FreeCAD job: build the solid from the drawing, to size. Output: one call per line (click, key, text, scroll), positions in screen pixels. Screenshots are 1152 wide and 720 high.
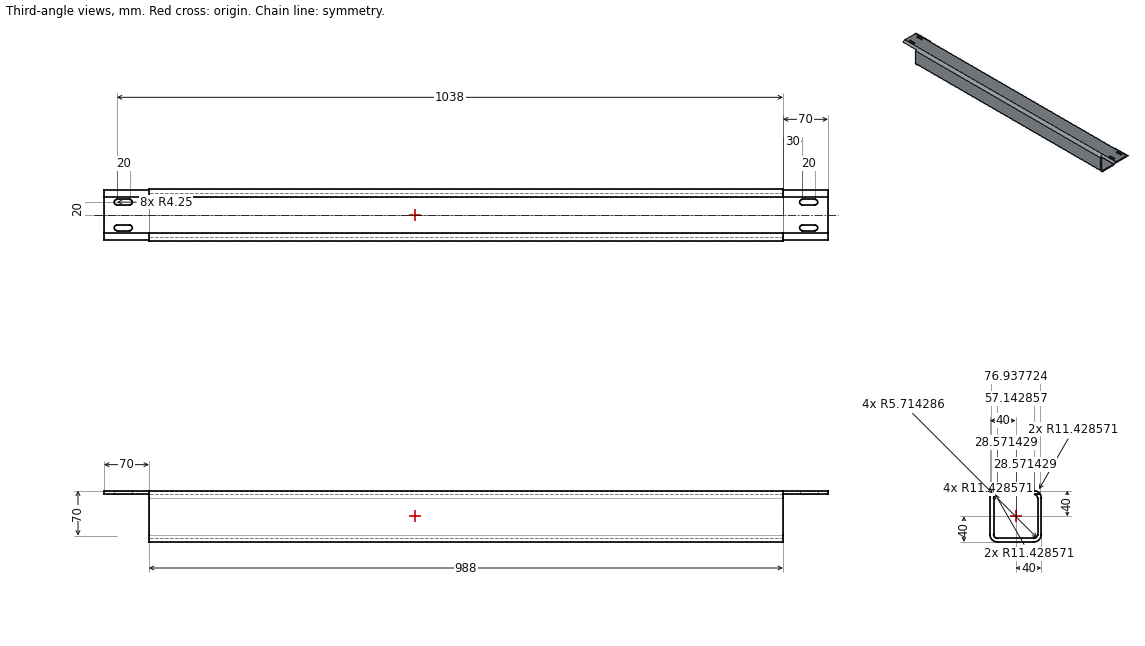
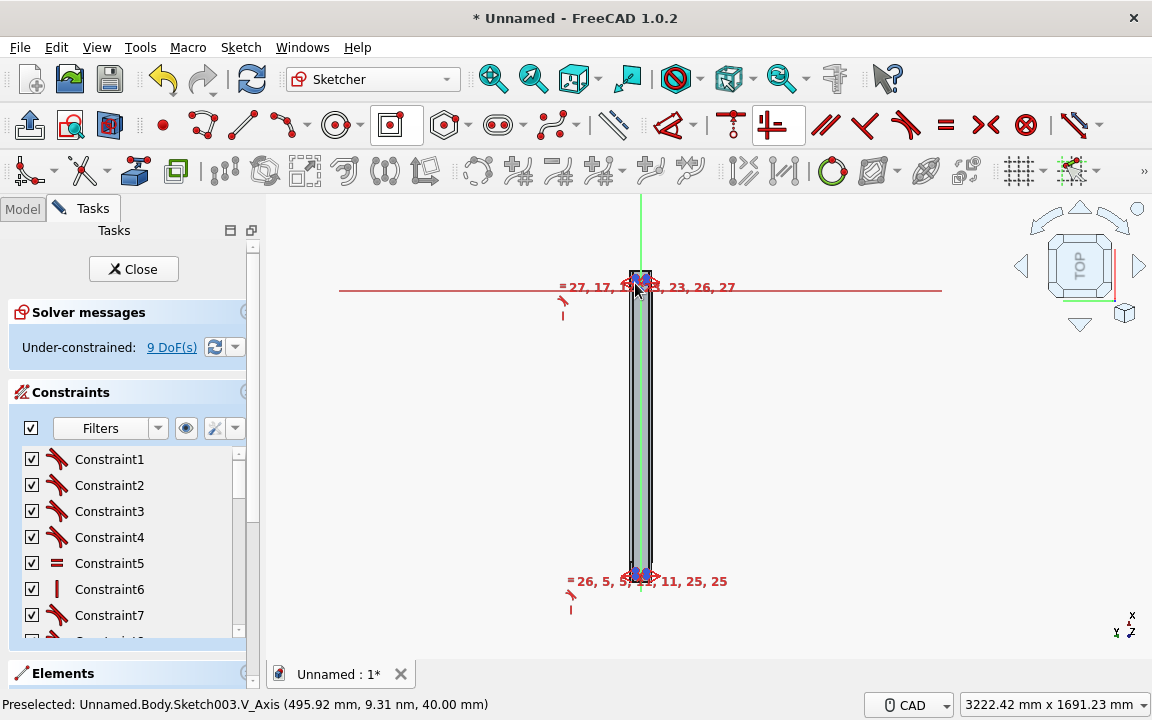
scroll(635, 577, up, 18)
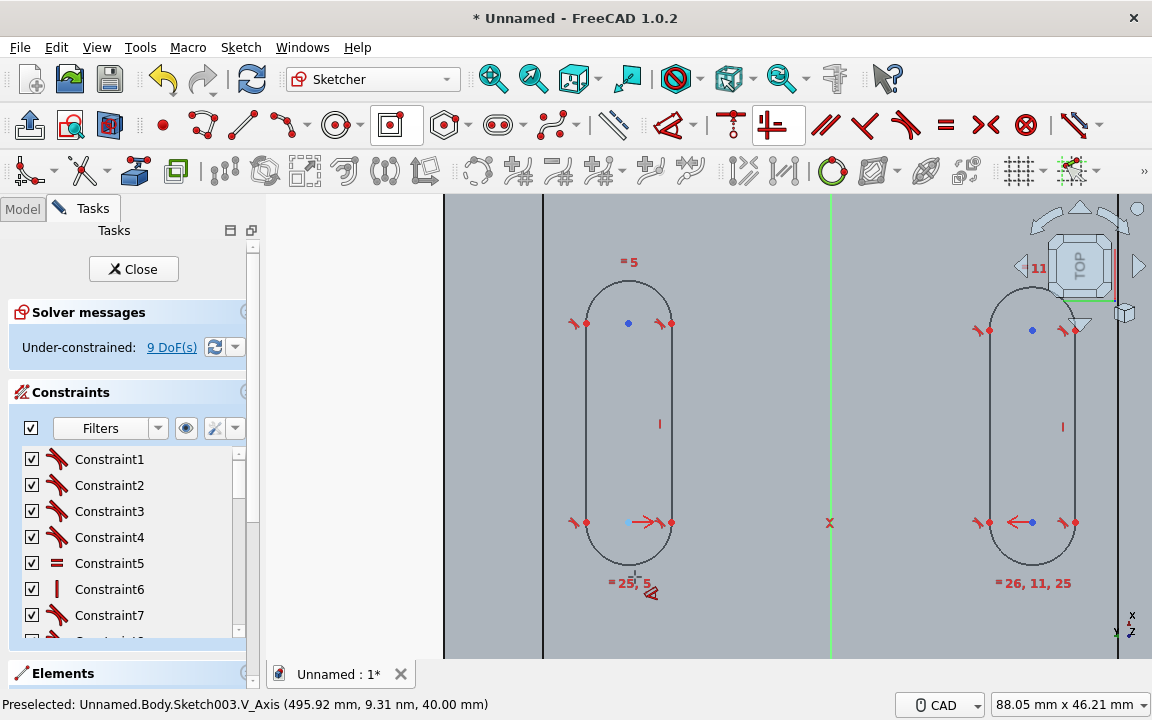
click(604, 557)
click(585, 583)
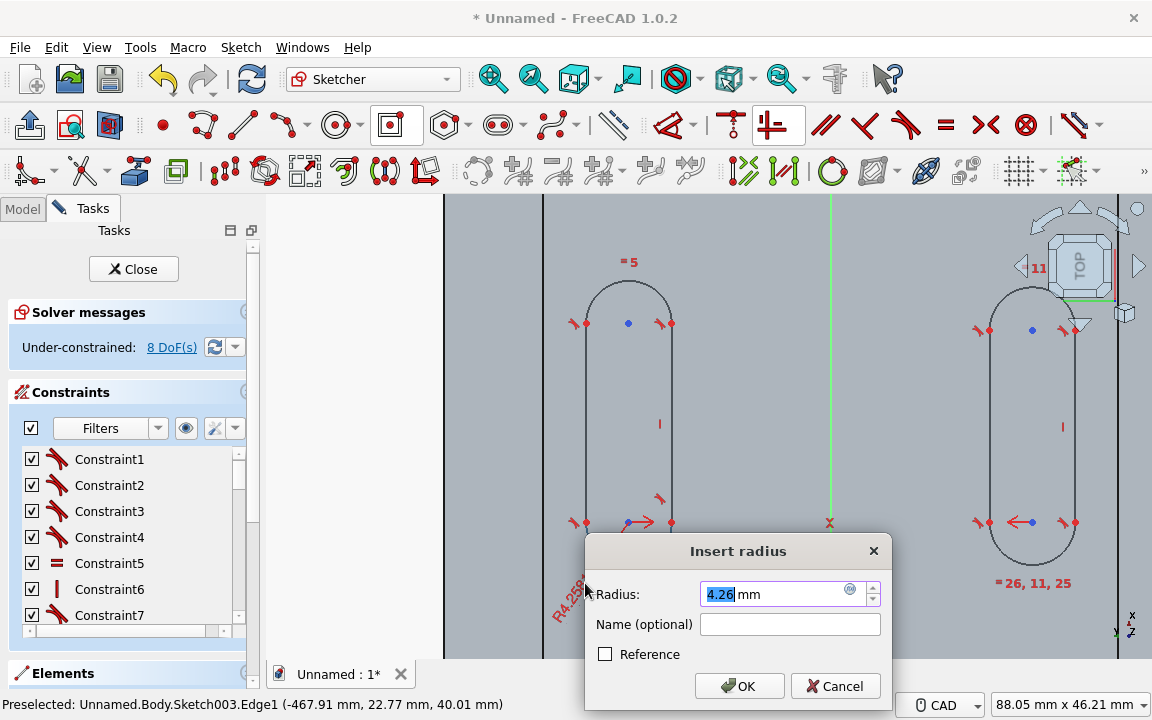
text(4.25)
key(Return)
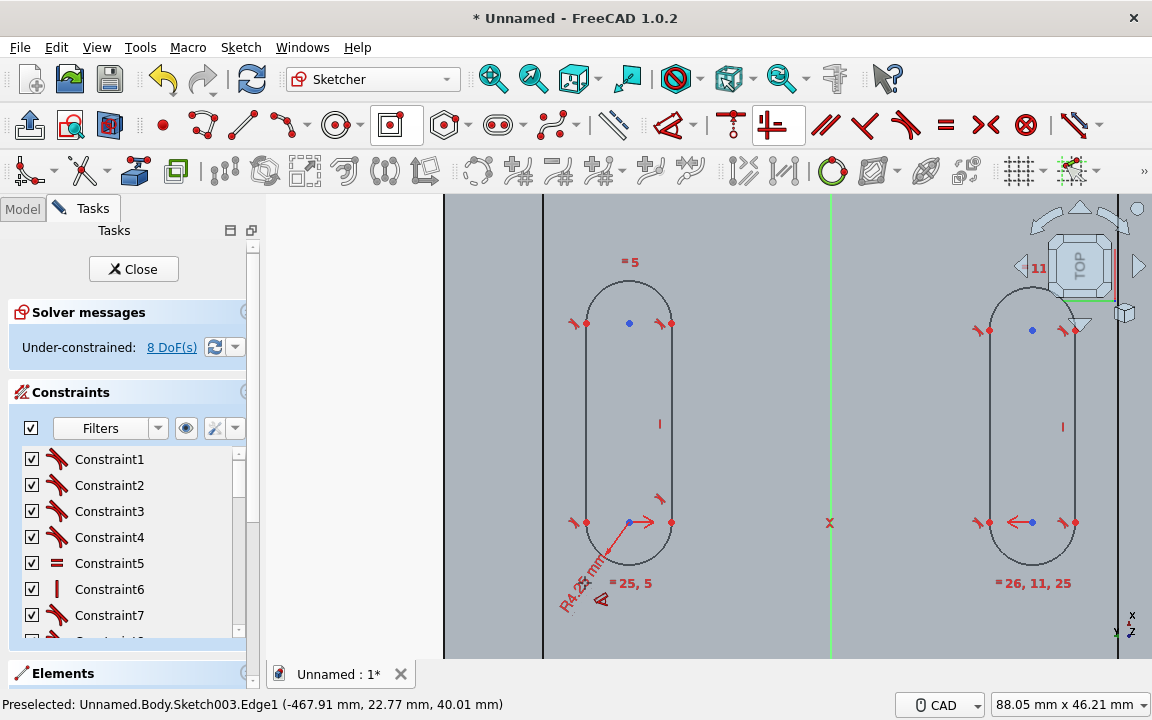
scroll(635, 578, down, 18)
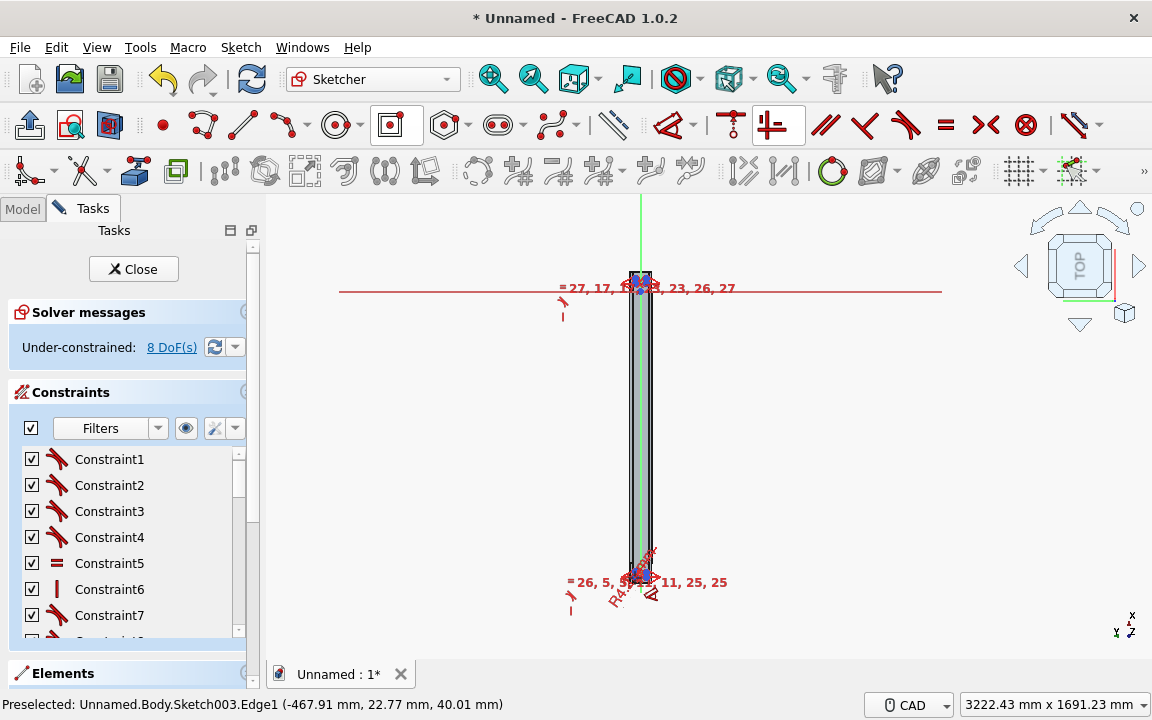
scroll(634, 576, up, 11)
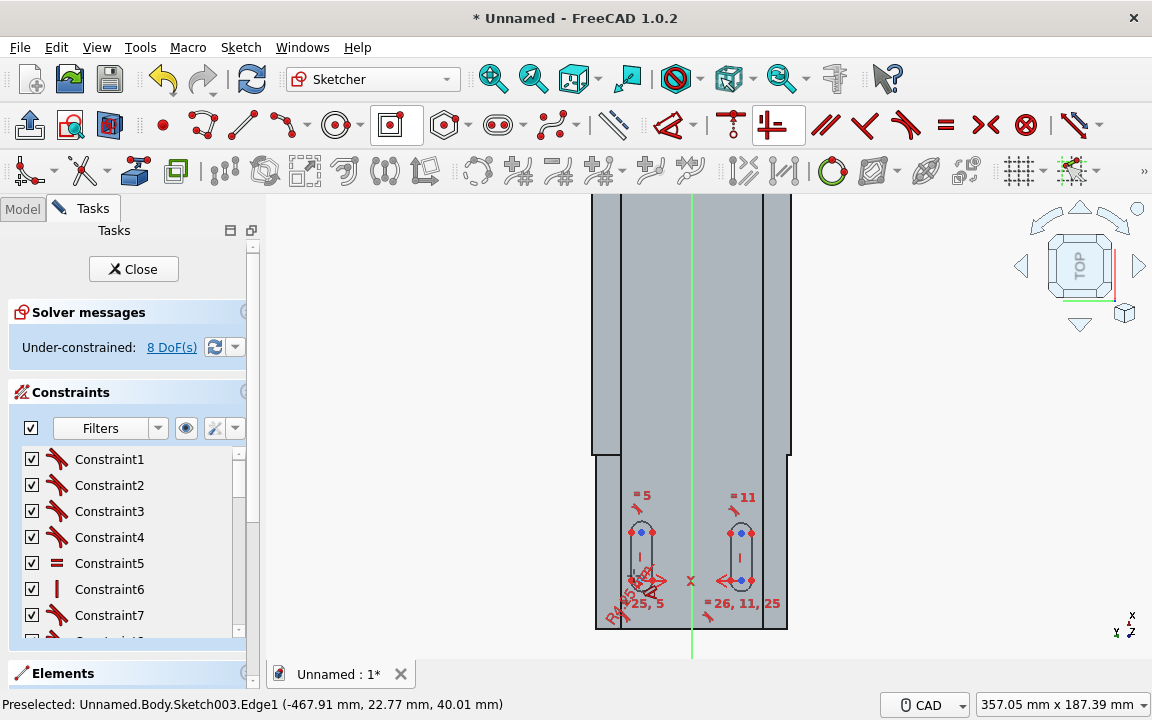
click(631, 566)
click(597, 556)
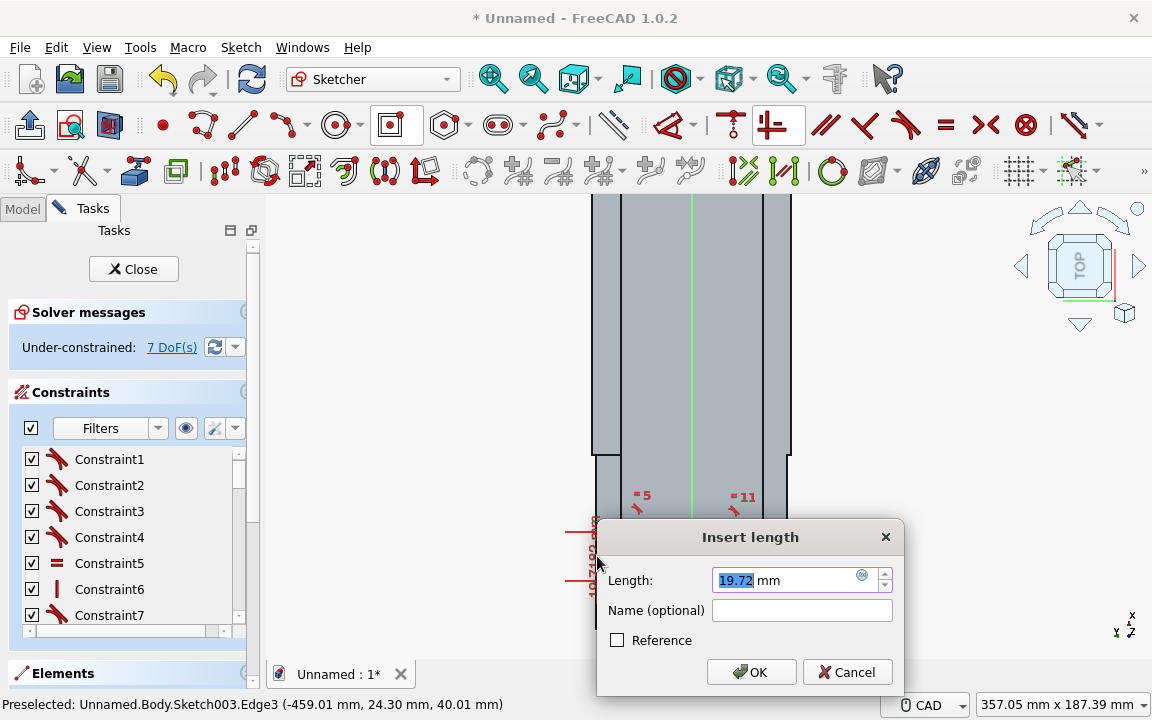
text(20)
key(Return)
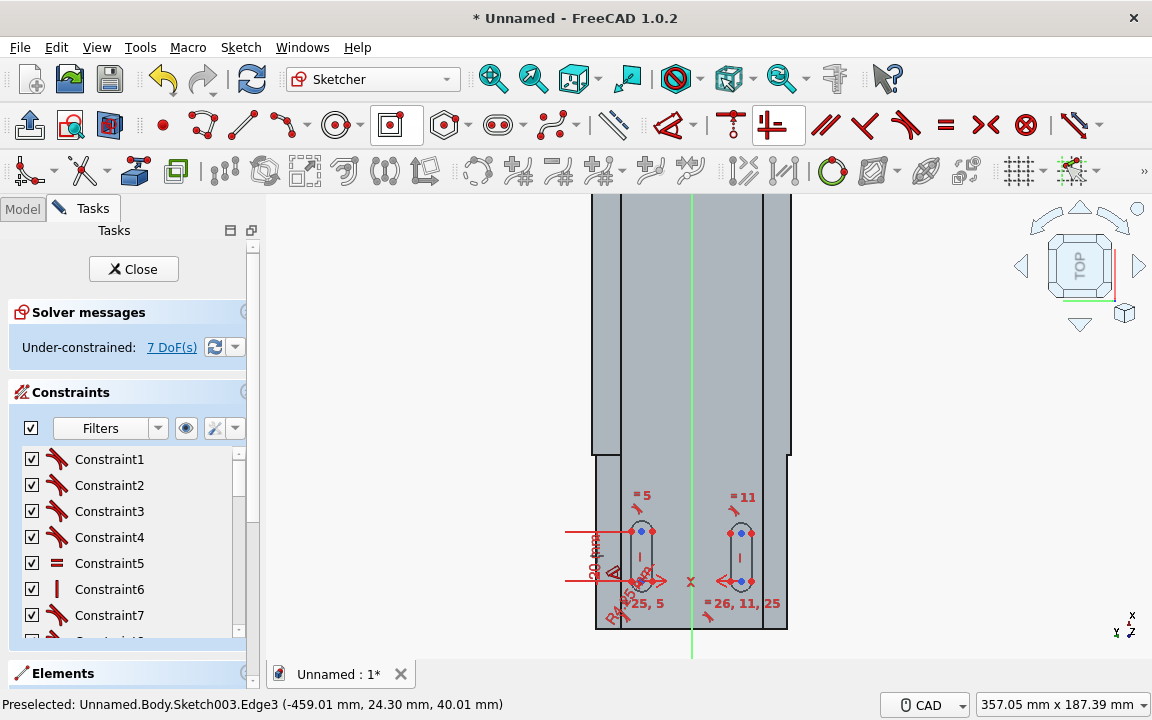
click(731, 567)
click(789, 557)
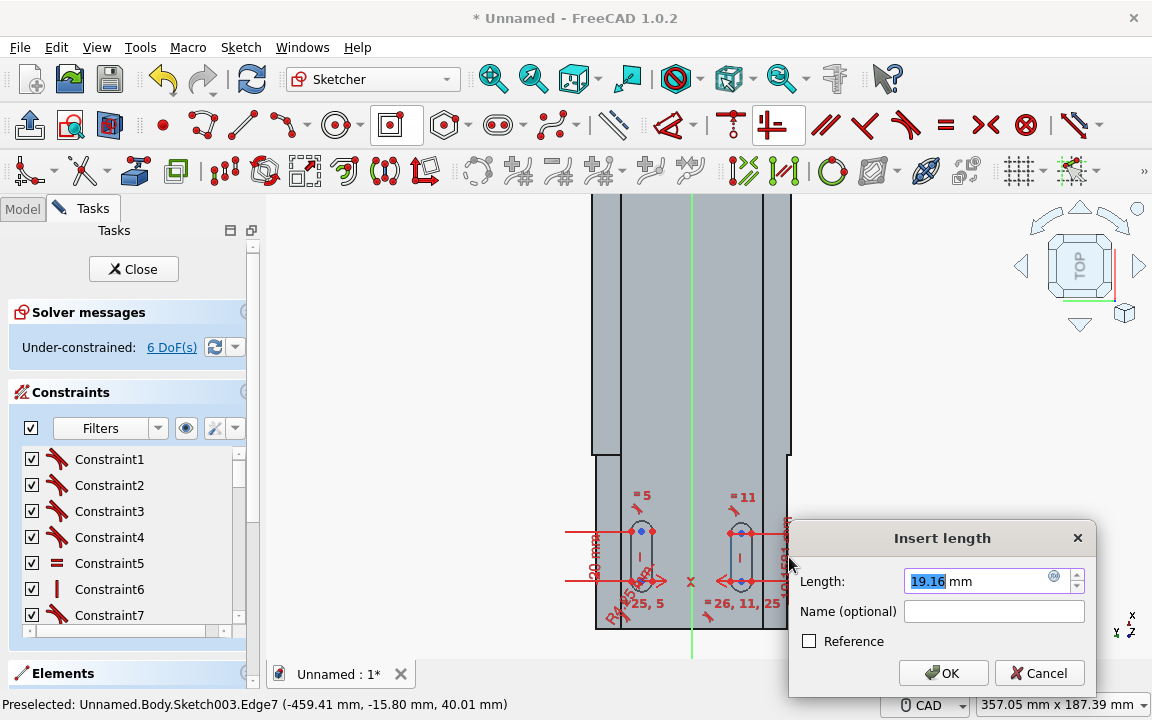
text(20)
key(Return)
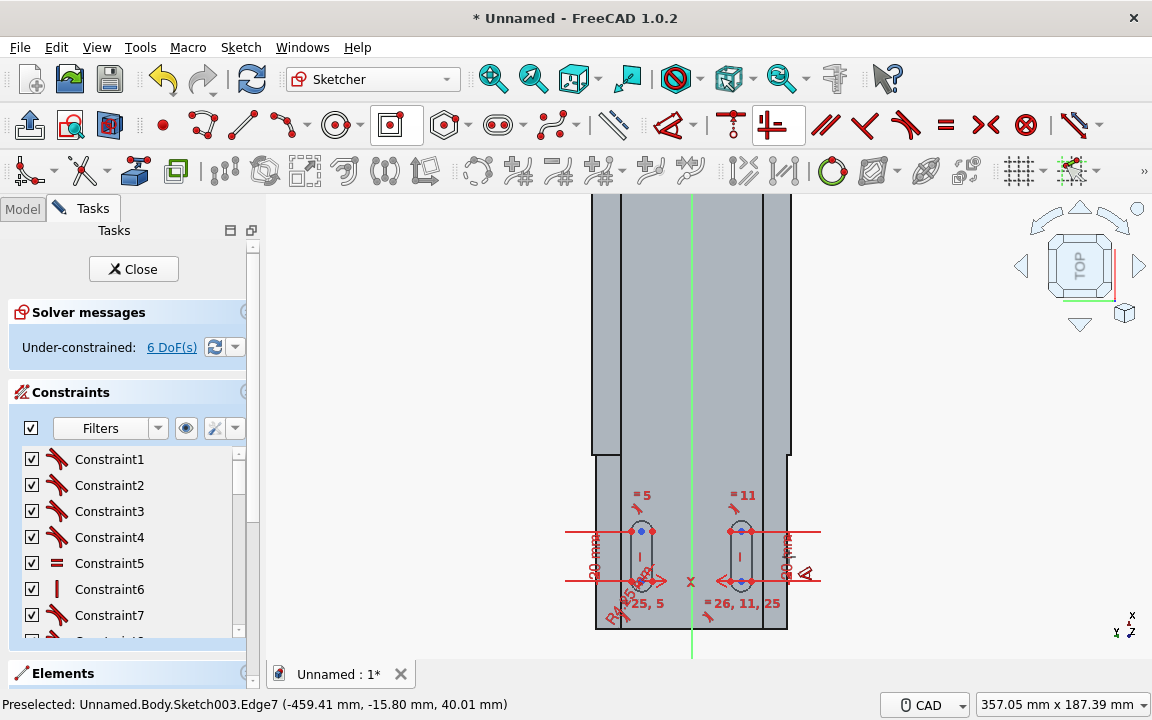
scroll(634, 576, down, 11)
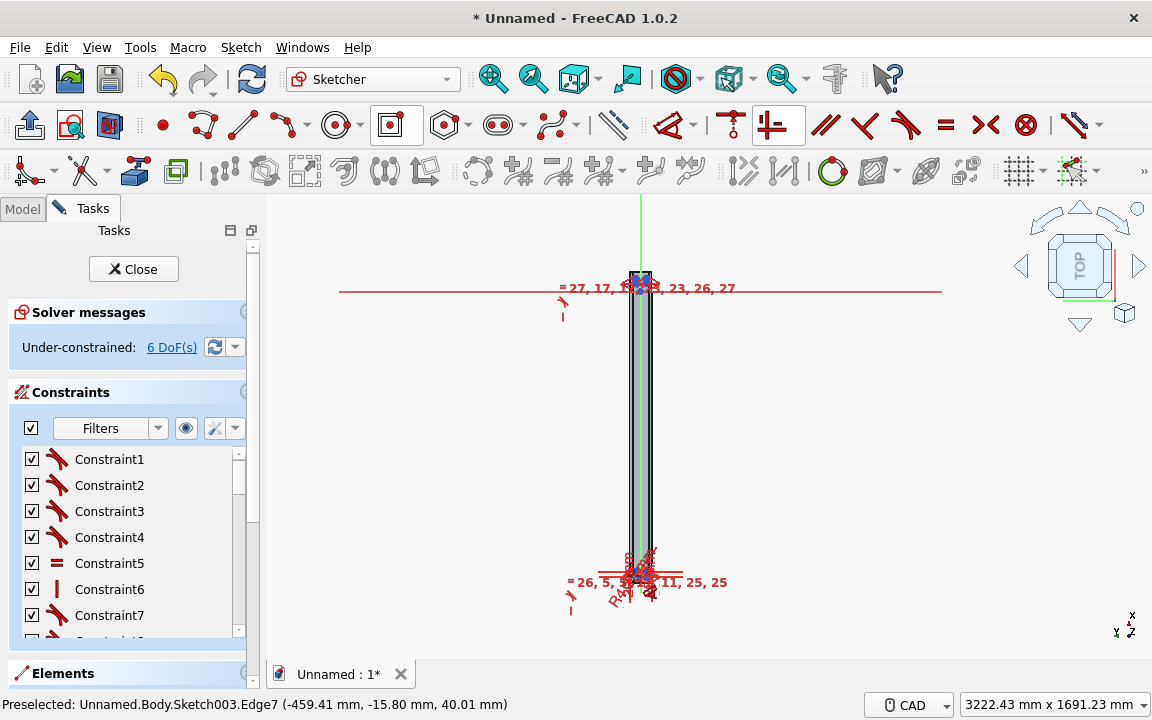
scroll(634, 282, up, 11)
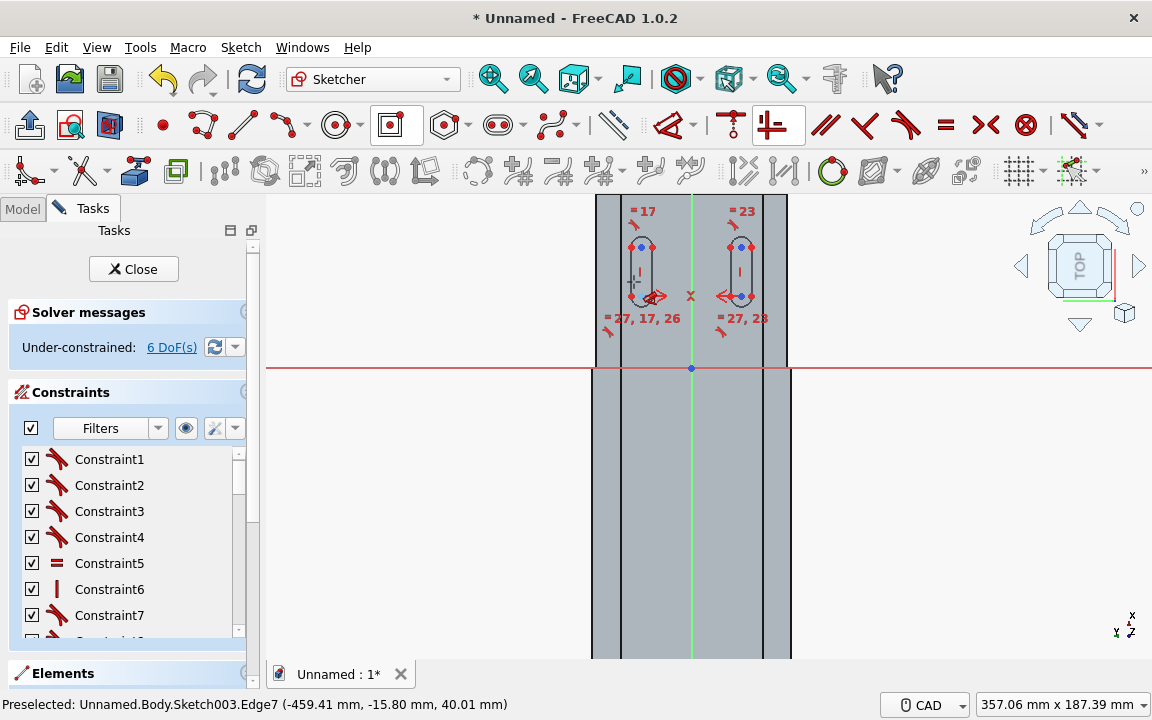
click(631, 282)
click(597, 272)